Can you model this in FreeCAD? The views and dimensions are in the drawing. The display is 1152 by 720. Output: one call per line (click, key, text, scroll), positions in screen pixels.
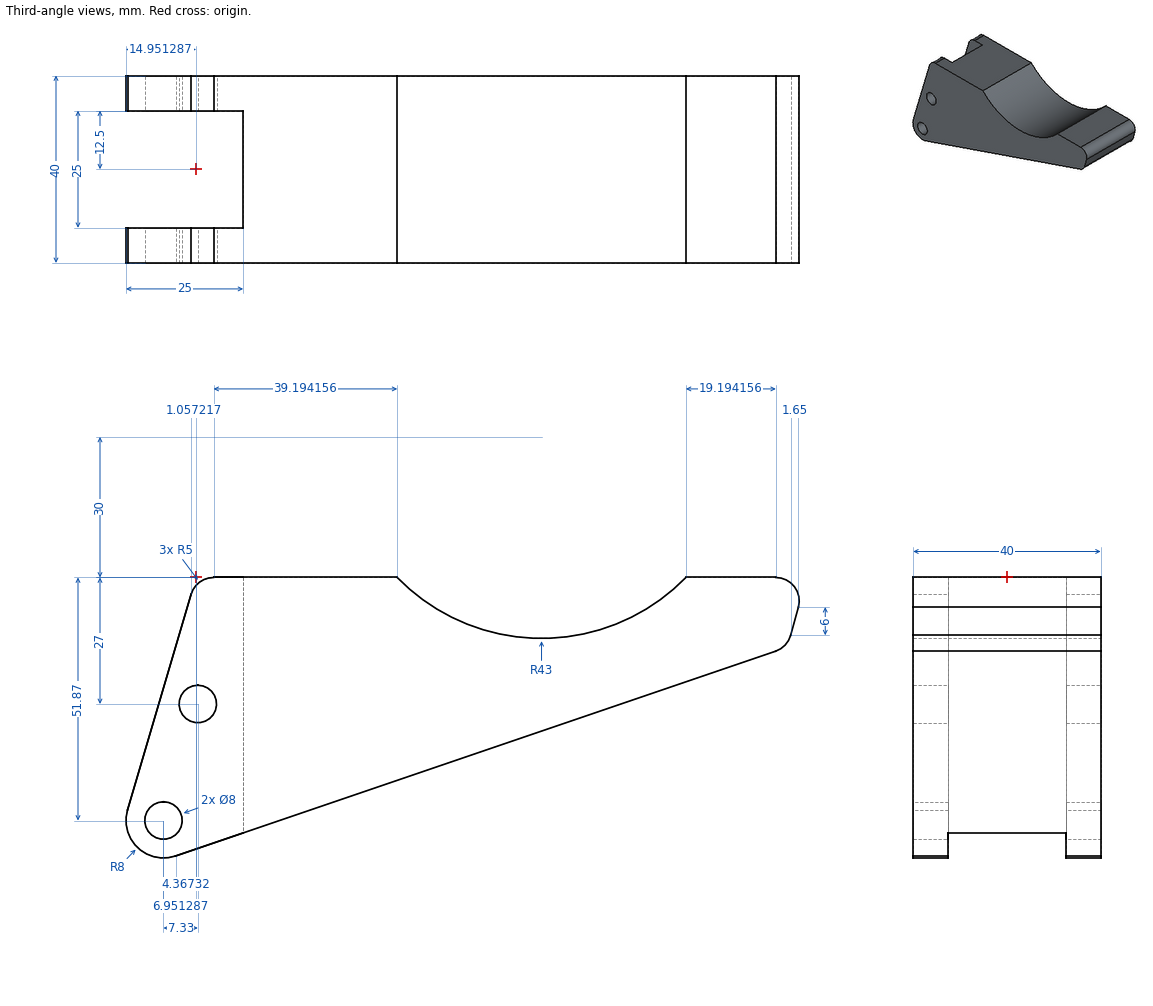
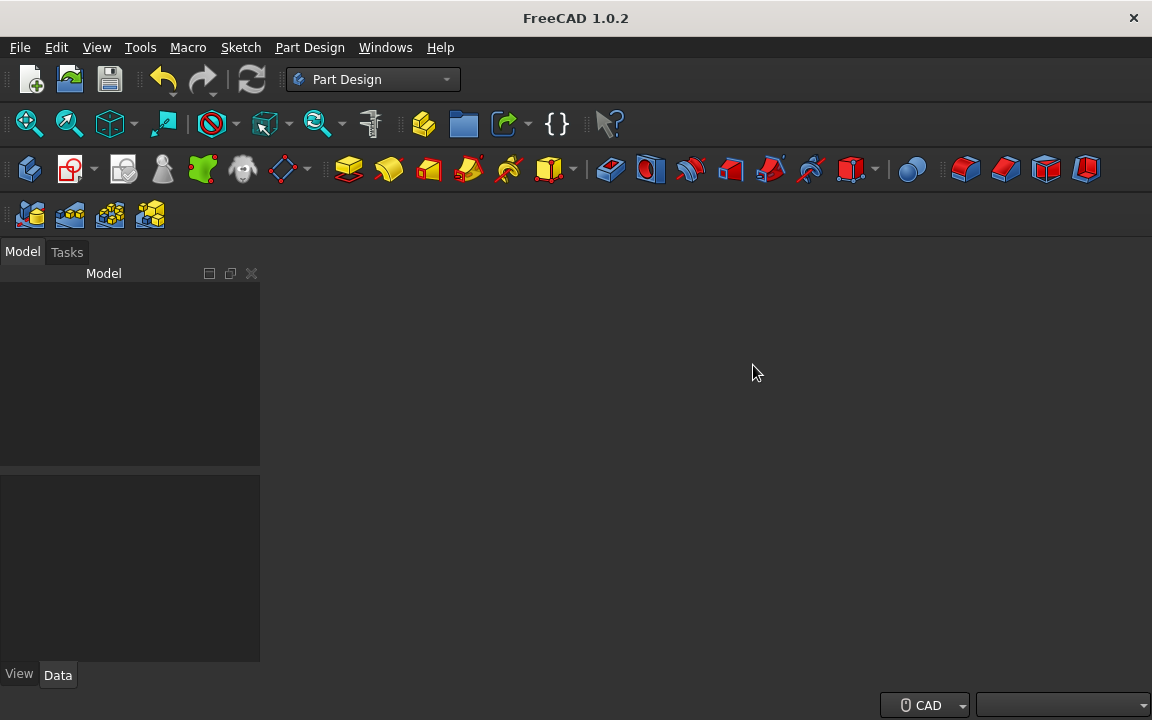
click(30, 80)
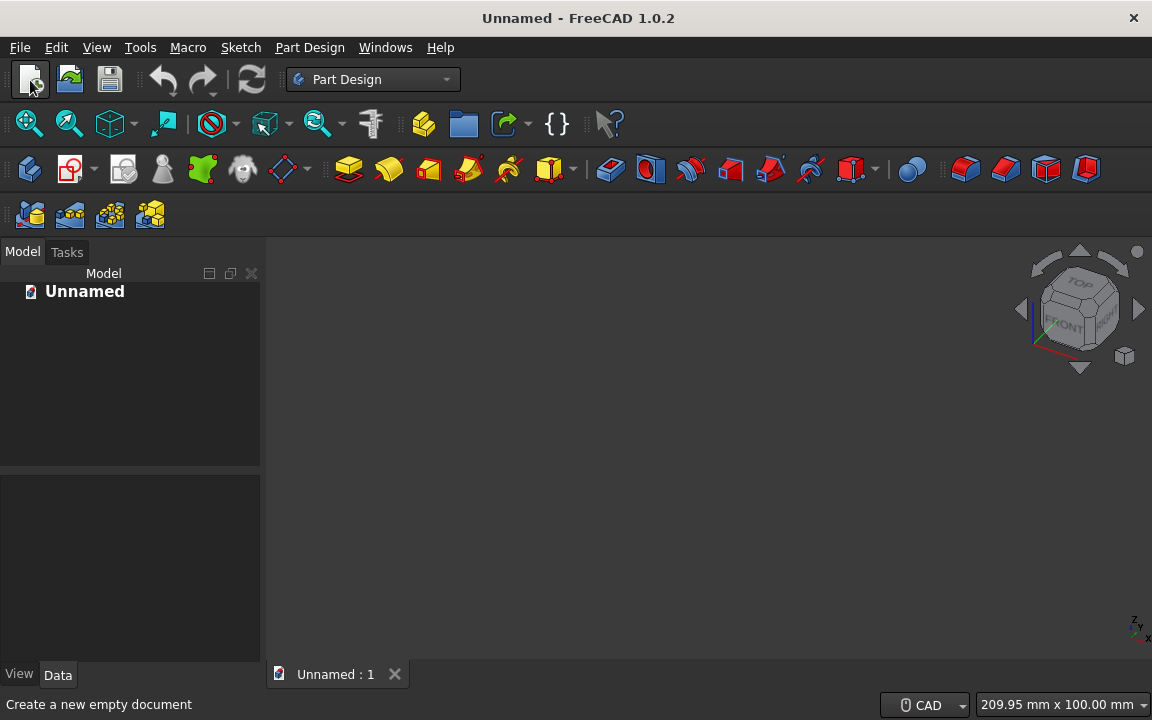
click(70, 170)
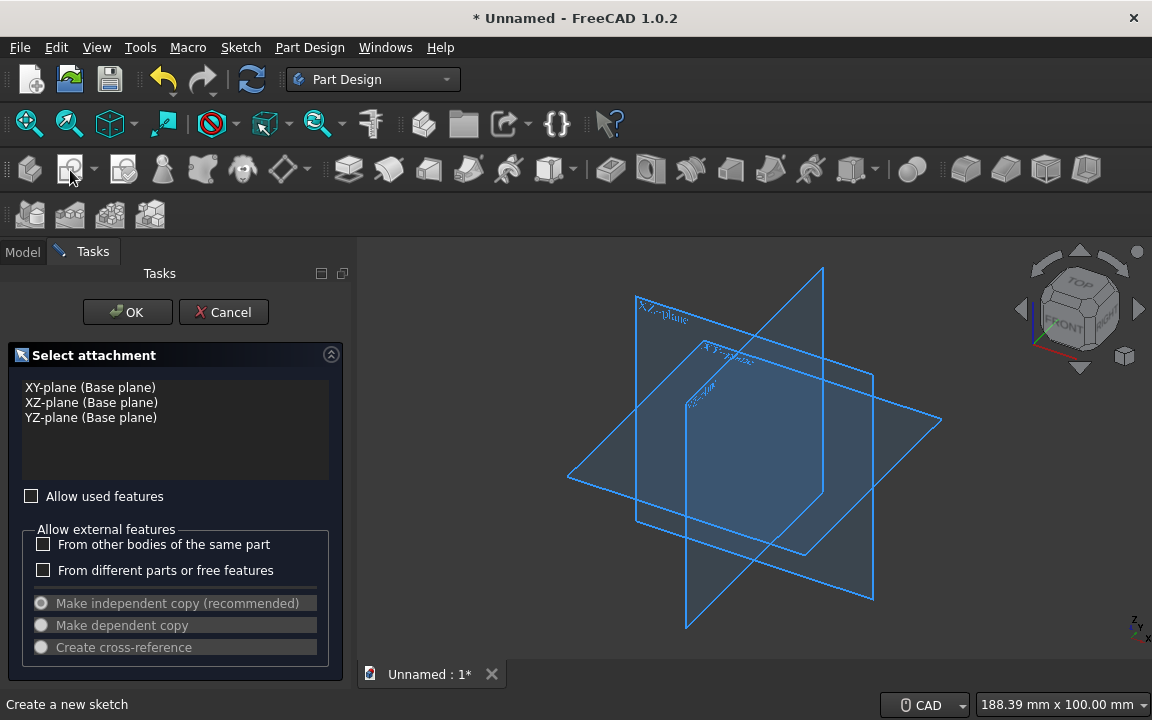
click(82, 402)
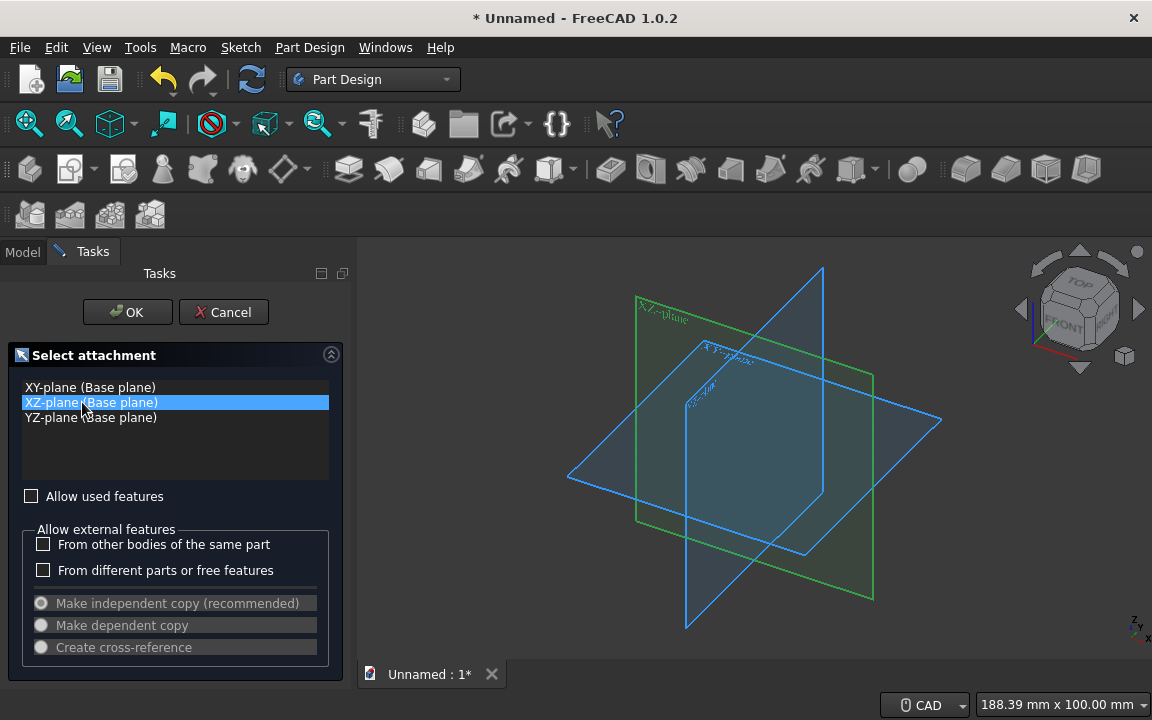
click(128, 312)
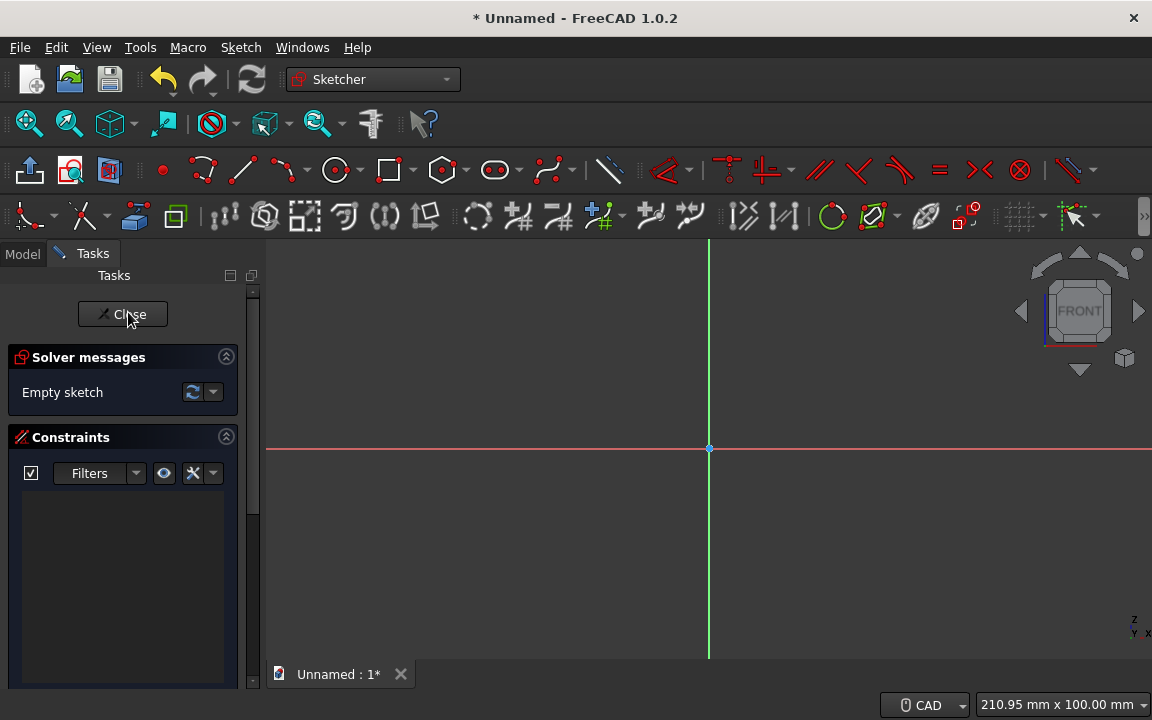
scroll(294, 267, down, 2)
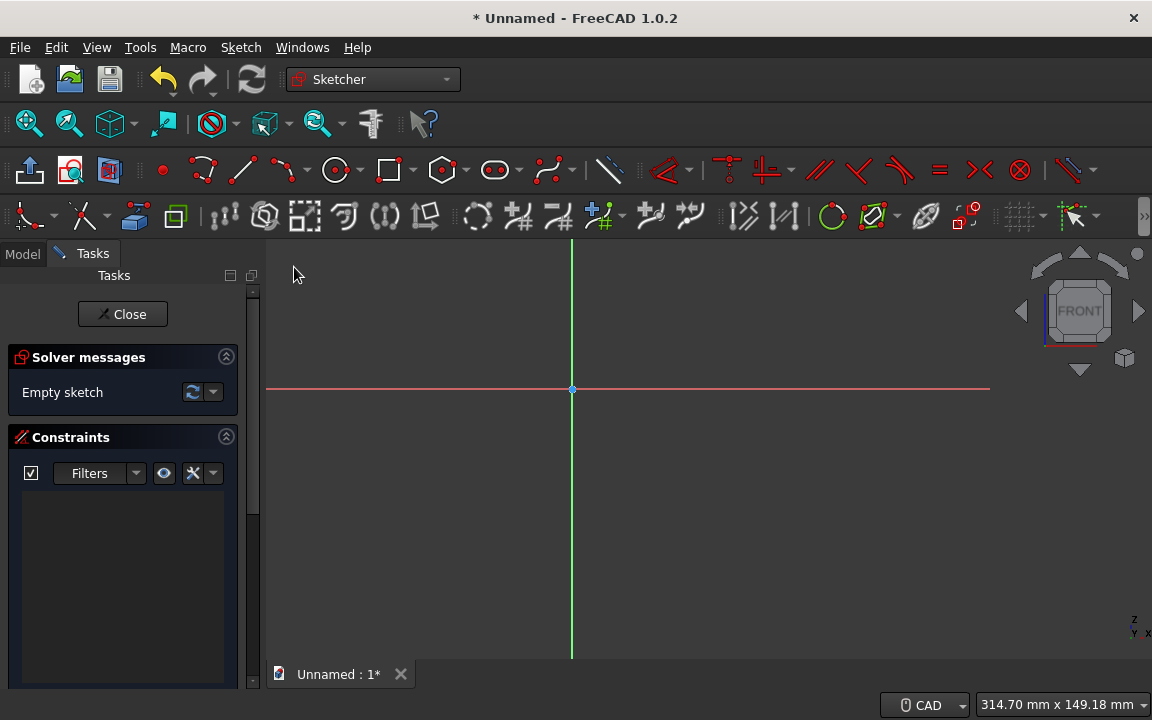
click(244, 170)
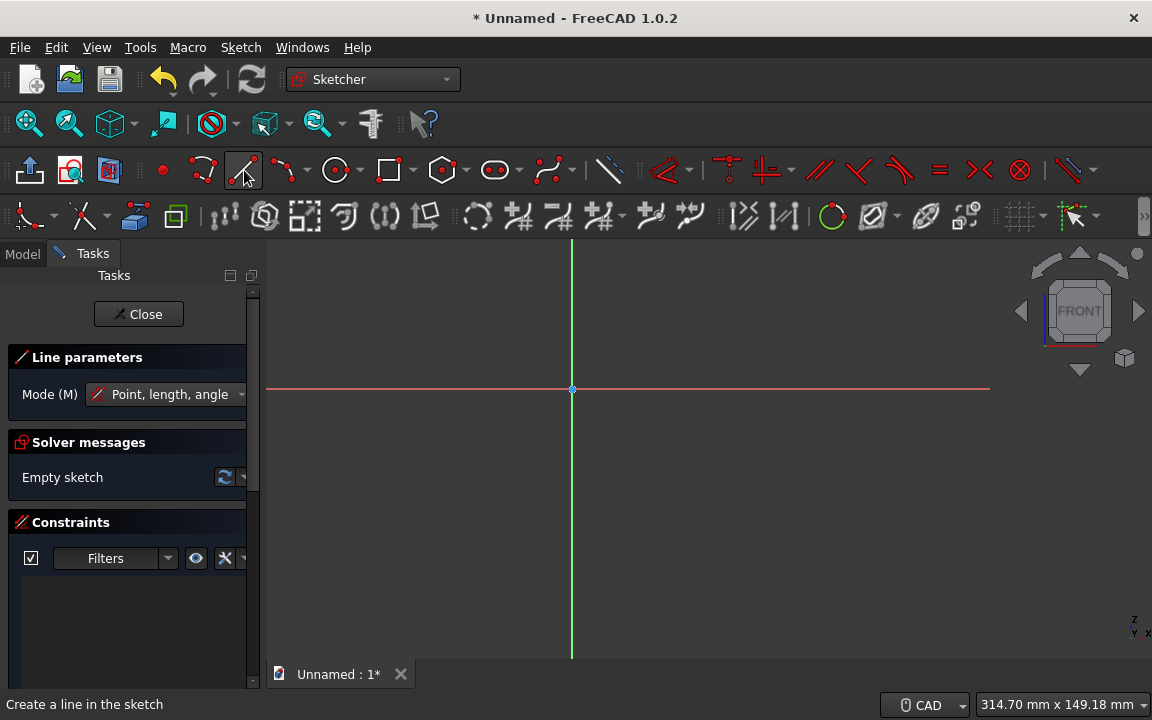
click(531, 529)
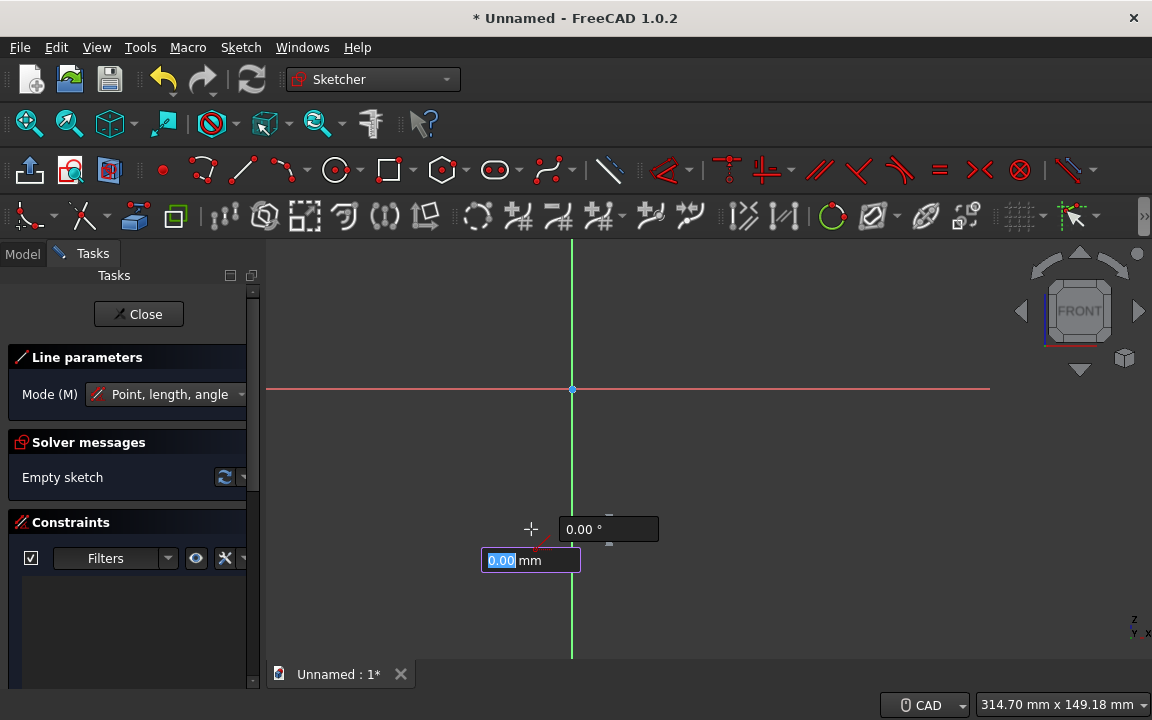
scroll(569, 399, up, 9)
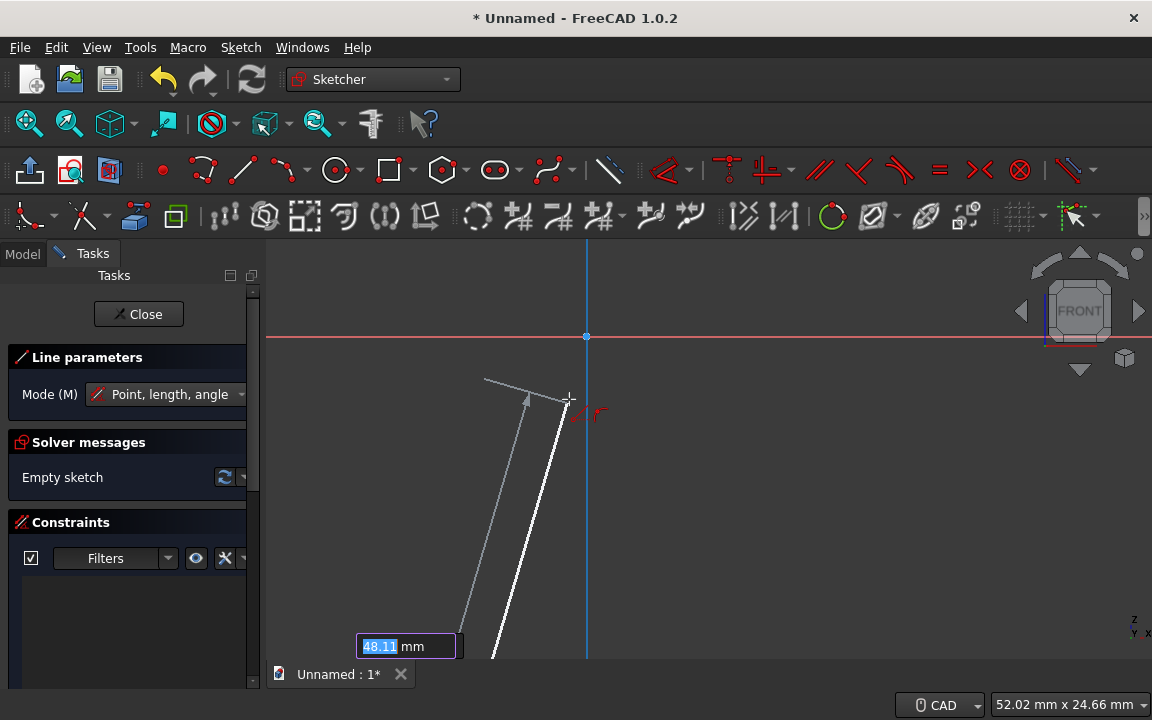
click(569, 398)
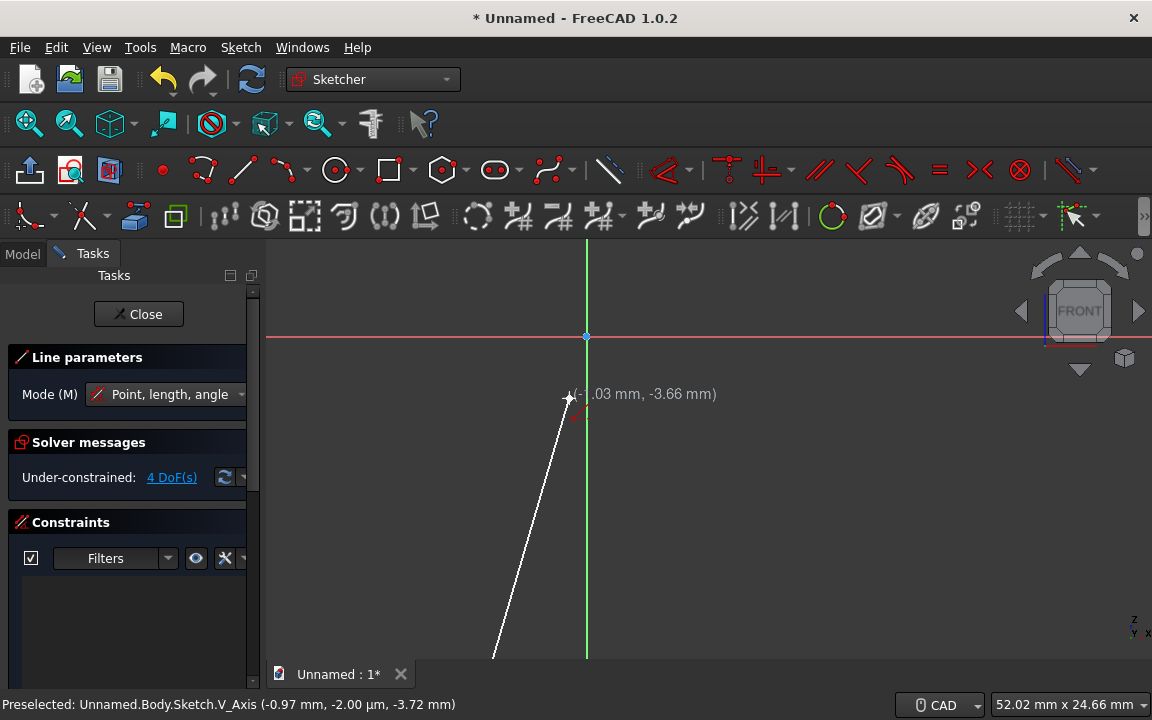
scroll(409, 349, down, 8)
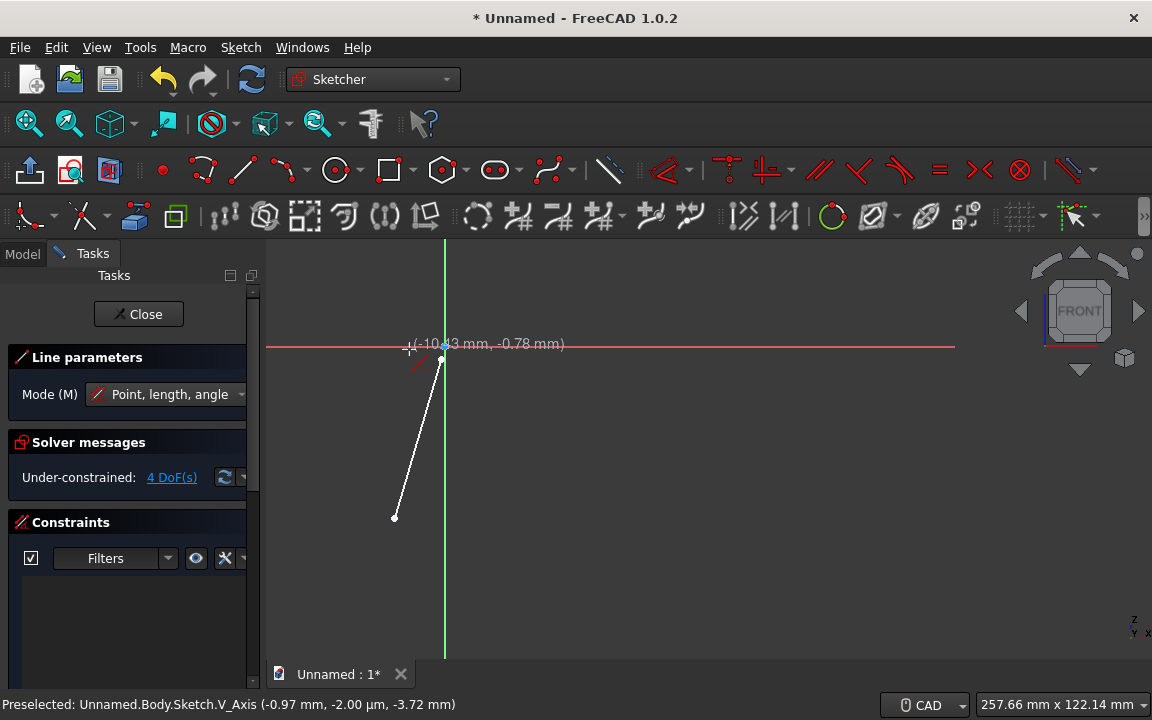
scroll(458, 347, up, 2)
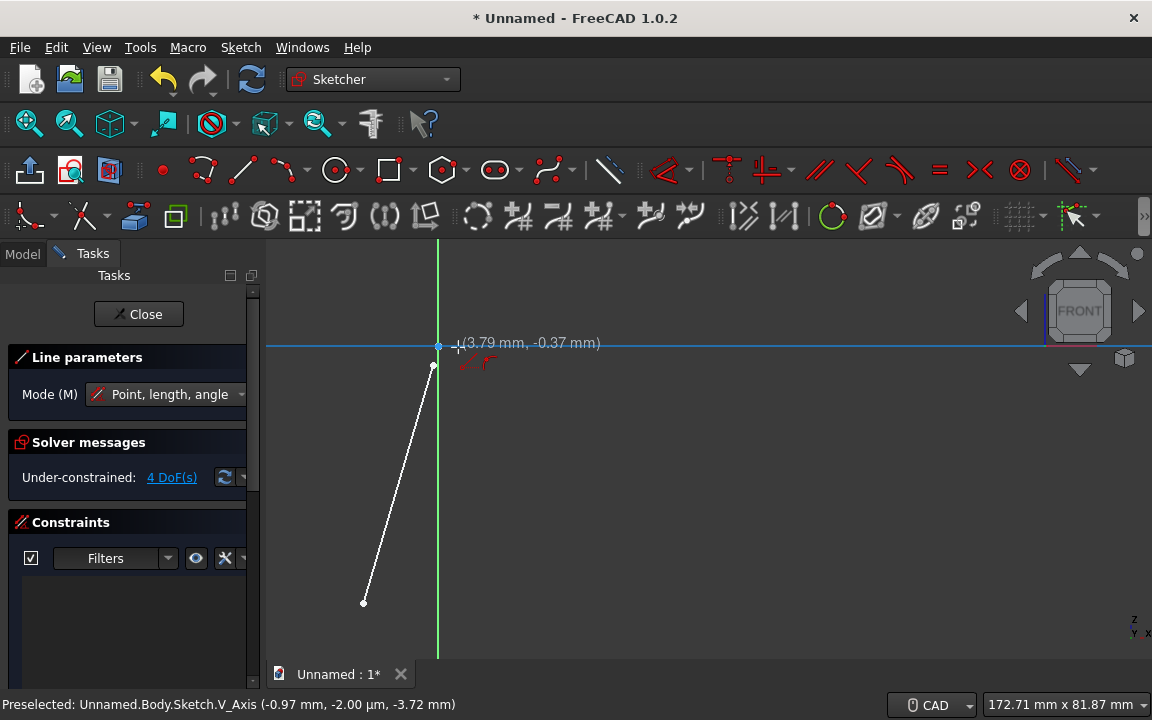
click(458, 346)
click(659, 355)